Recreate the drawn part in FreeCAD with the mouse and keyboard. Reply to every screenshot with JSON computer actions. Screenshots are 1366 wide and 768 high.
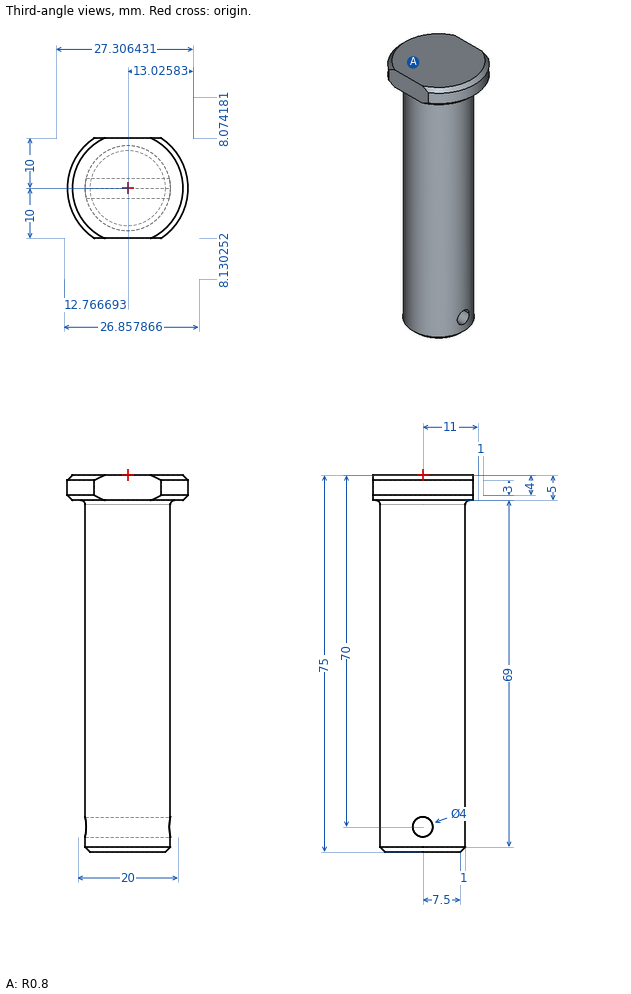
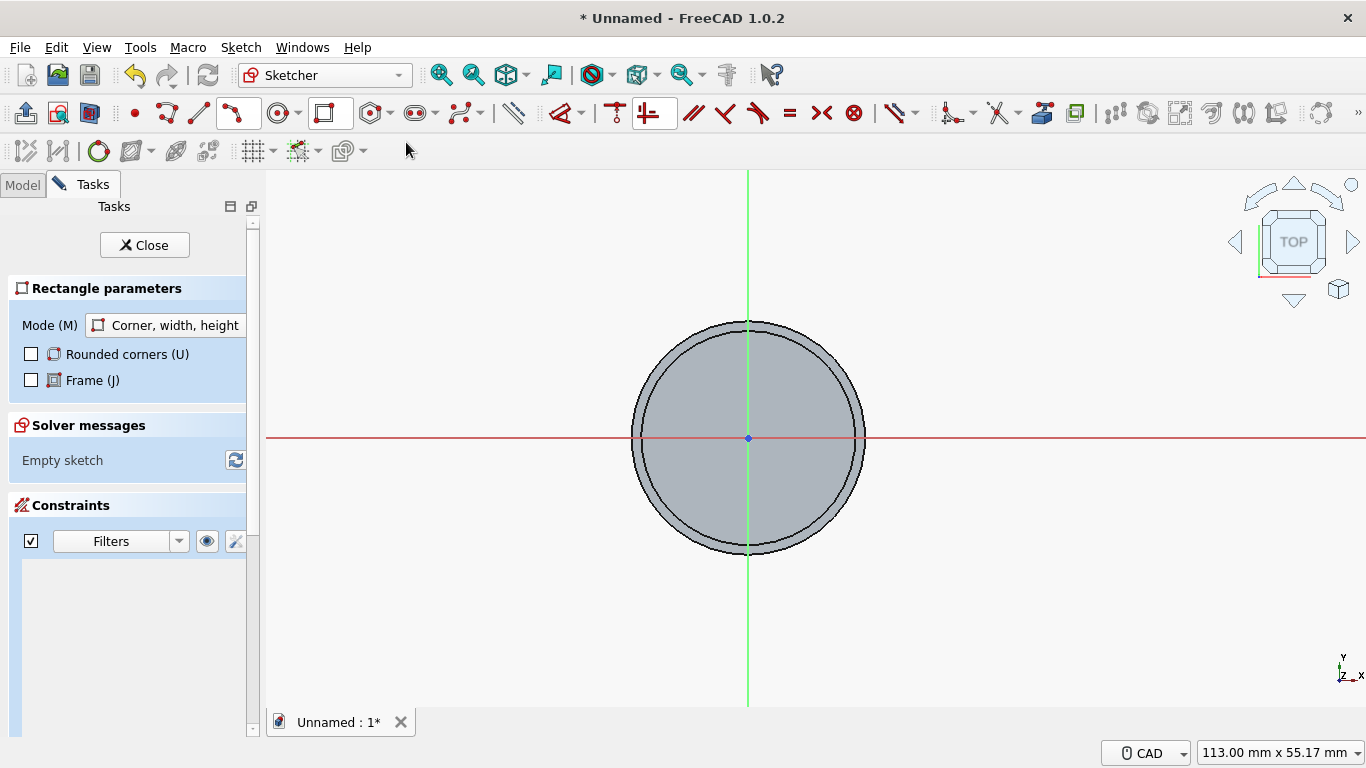
{"action": "left_click", "coordinate": [609, 262]}
{"action": "mouse_move", "coordinate": [875, 341]}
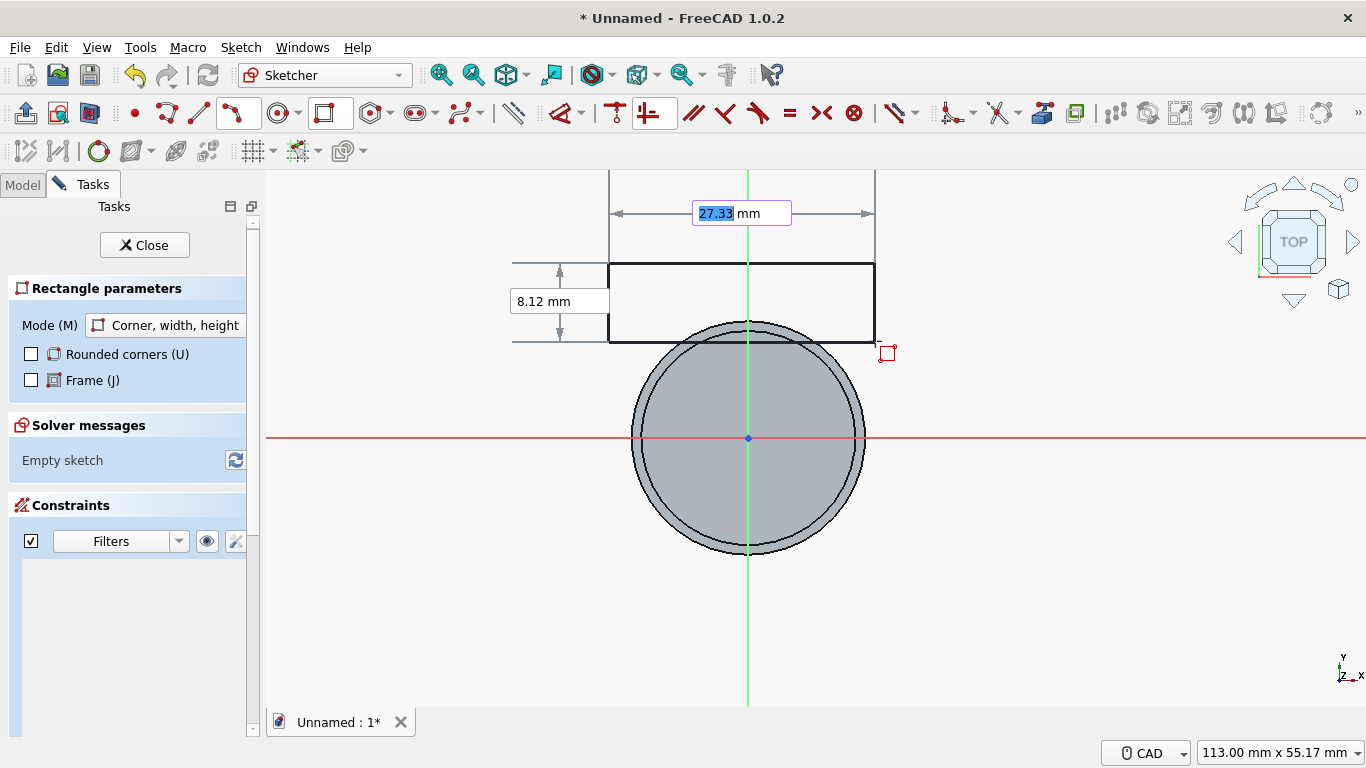
{"action": "type", "text": "27.306431"}
{"action": "key", "text": "Tab"}
{"action": "type", "text": "8.074181"}
{"action": "key", "text": "Return"}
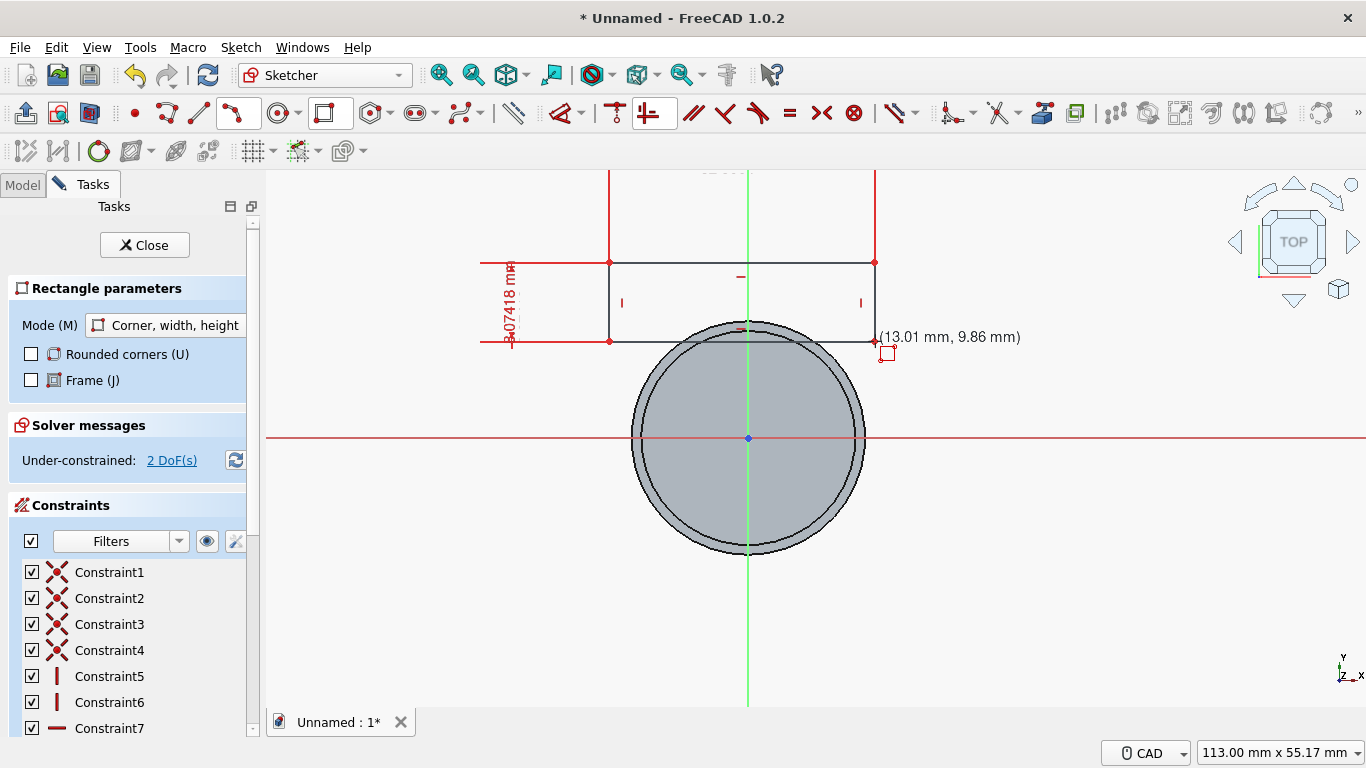
{"action": "left_click", "coordinate": [624, 535]}
{"action": "mouse_move", "coordinate": [885, 614]}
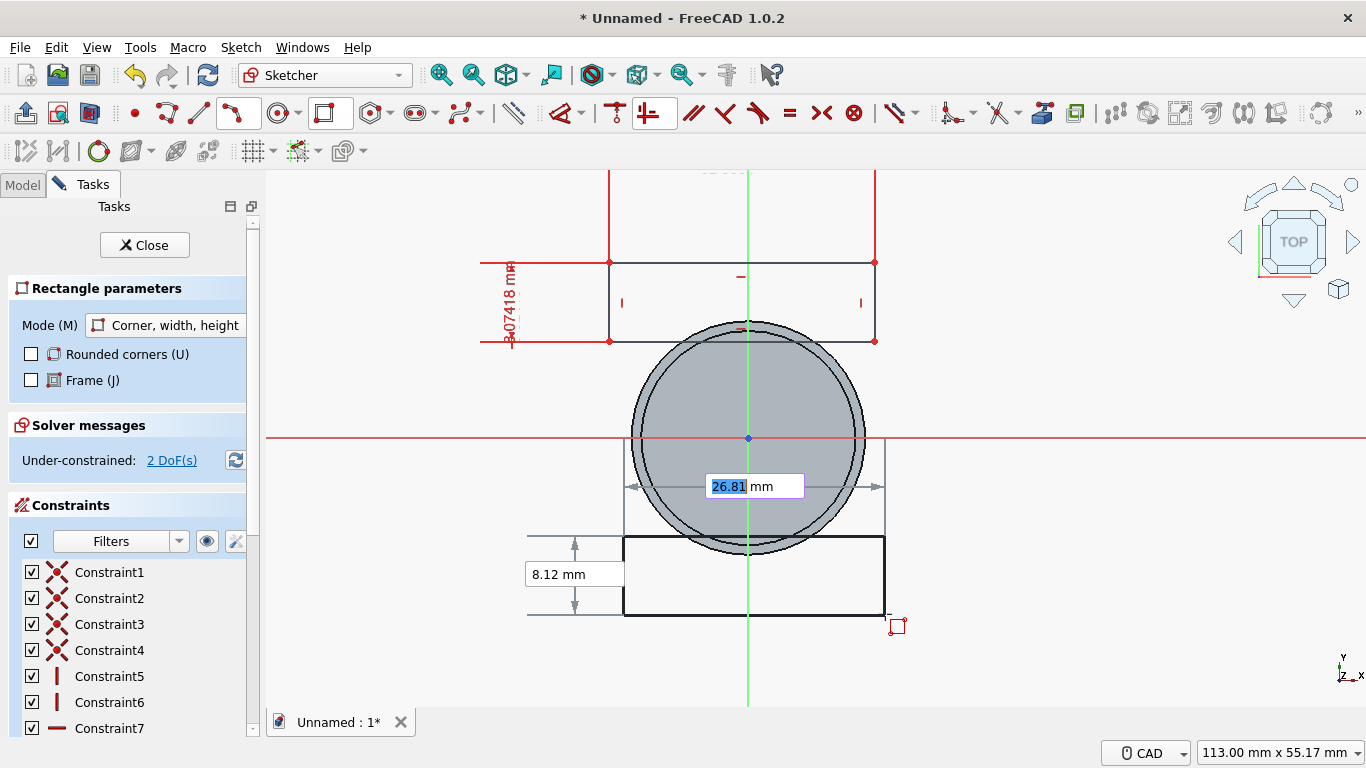
{"action": "type", "text": "26.857866"}
{"action": "key", "text": "Tab"}
{"action": "type", "text": "8.130252"}
{"action": "key", "text": "Return"}
{"action": "key", "text": "Escape"}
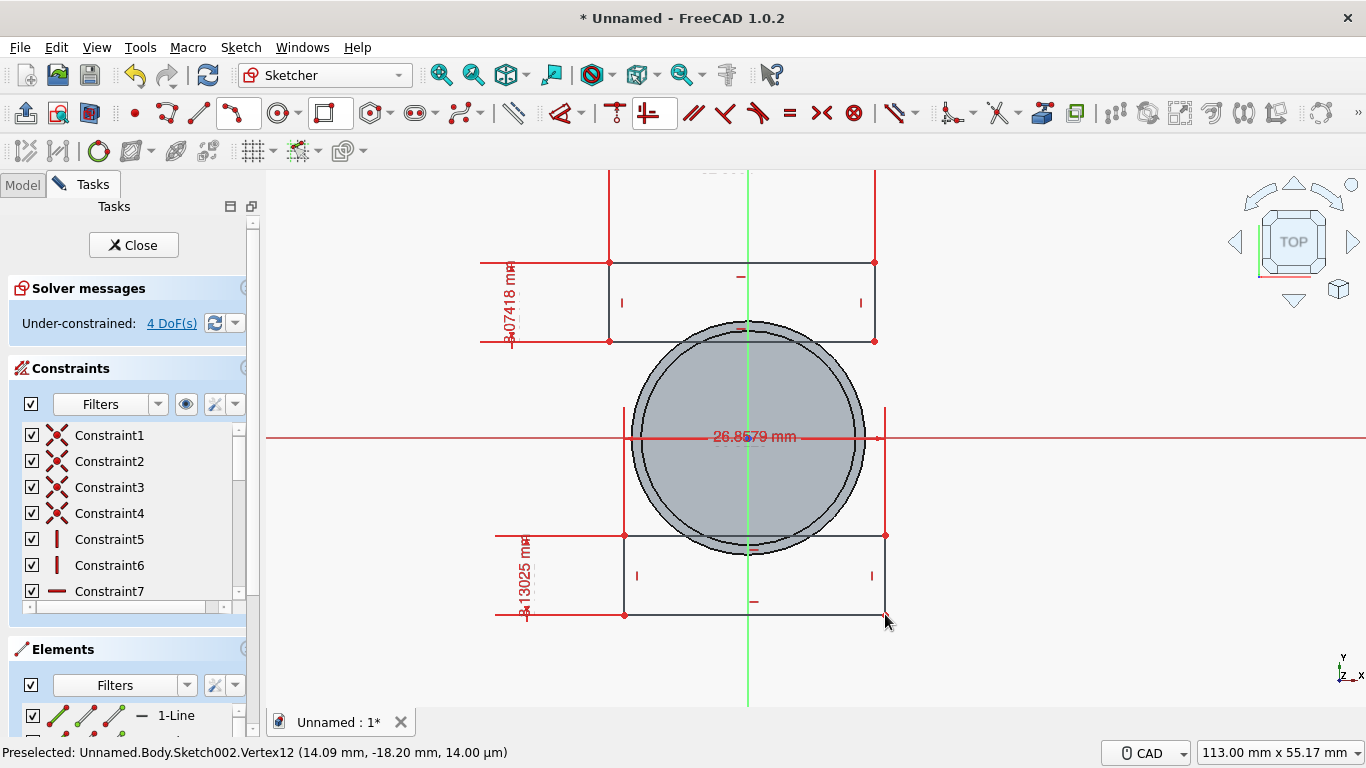
{"action": "left_click", "coordinate": [560, 114]}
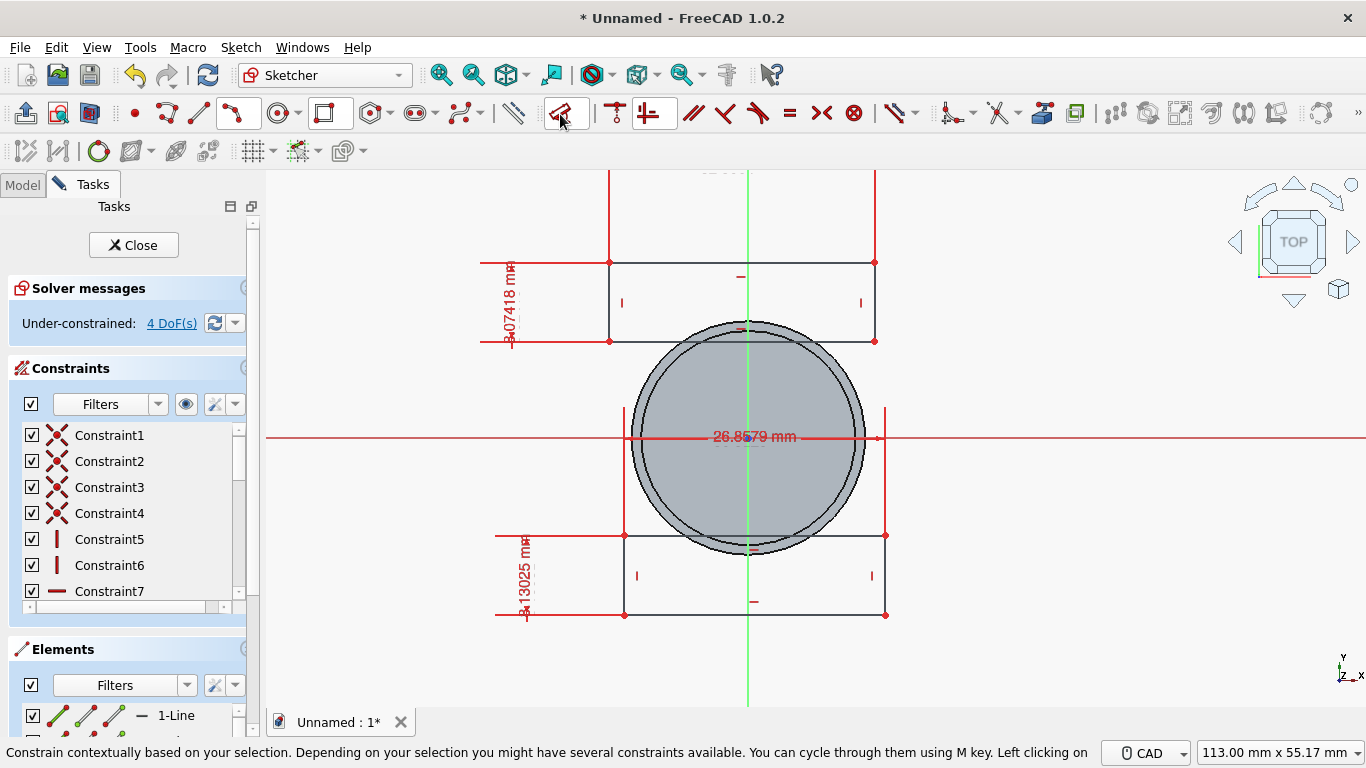
{"action": "left_click", "coordinate": [609, 342]}
{"action": "left_click", "coordinate": [575, 390]}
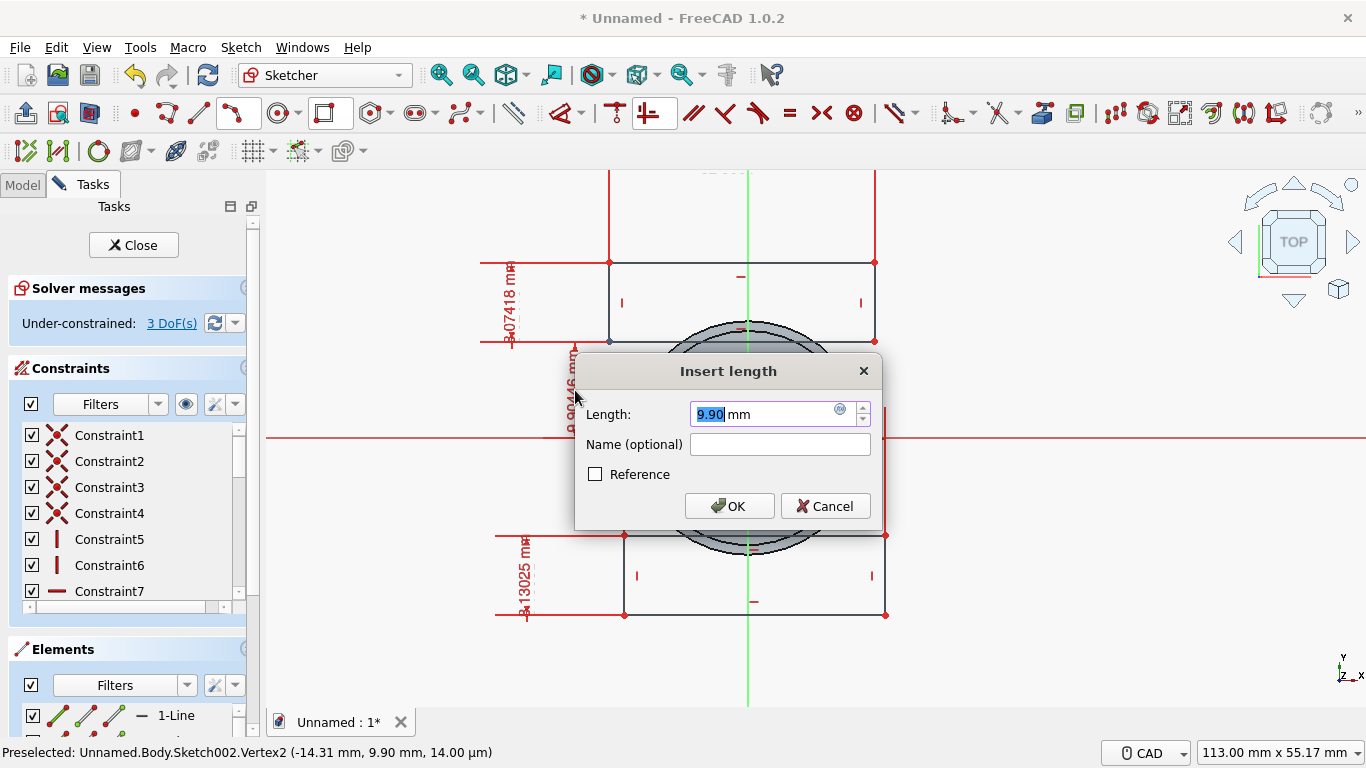
{"action": "type", "text": "10"}
{"action": "key", "text": "Return"}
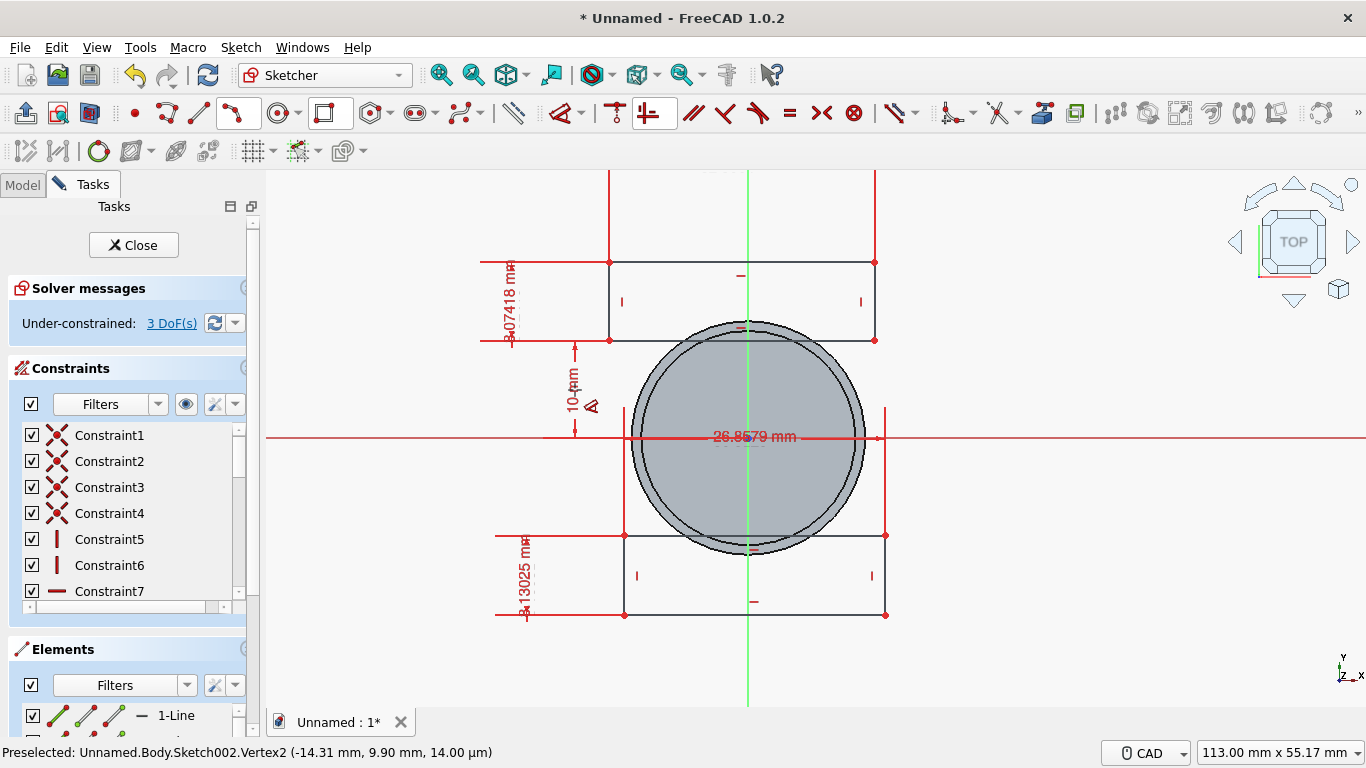
{"action": "left_click", "coordinate": [624, 536]}
{"action": "left_click", "coordinate": [590, 487]}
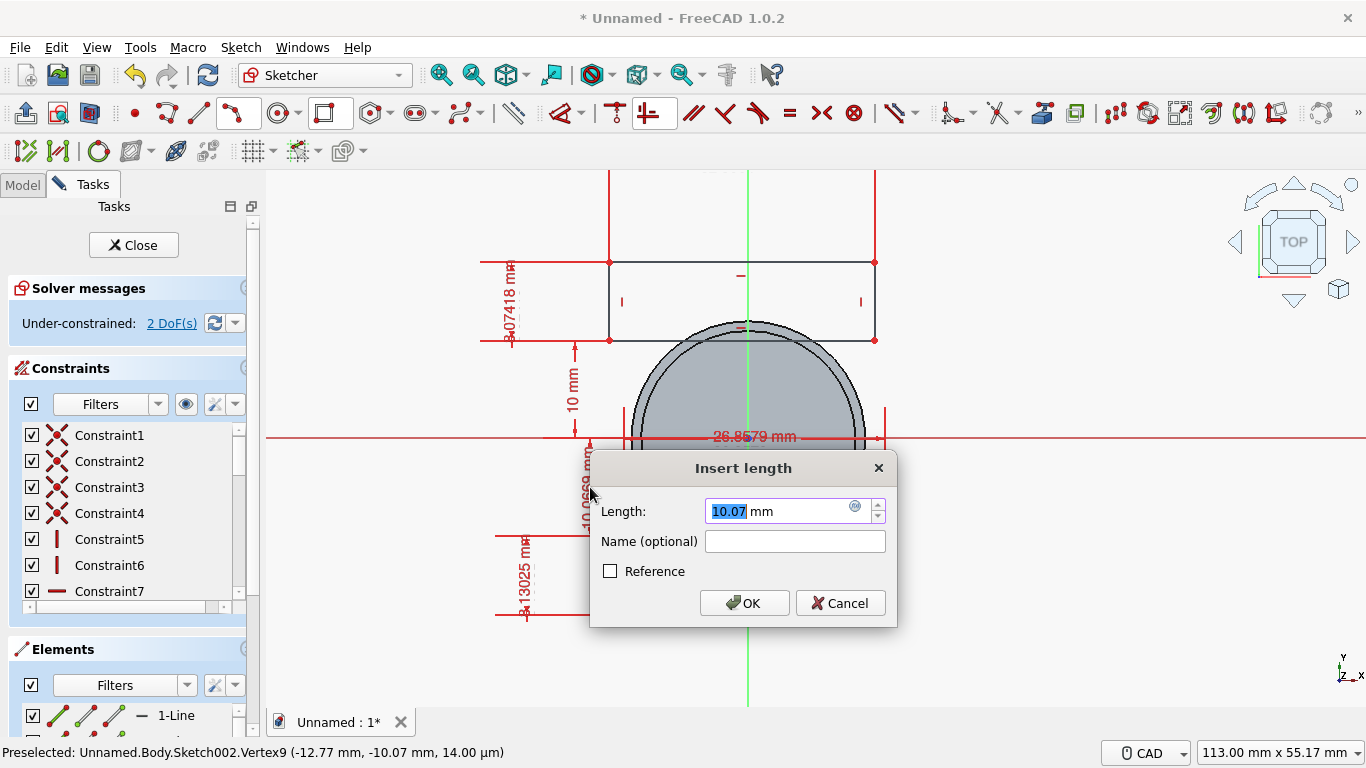
{"action": "type", "text": "10"}
{"action": "key", "text": "Return"}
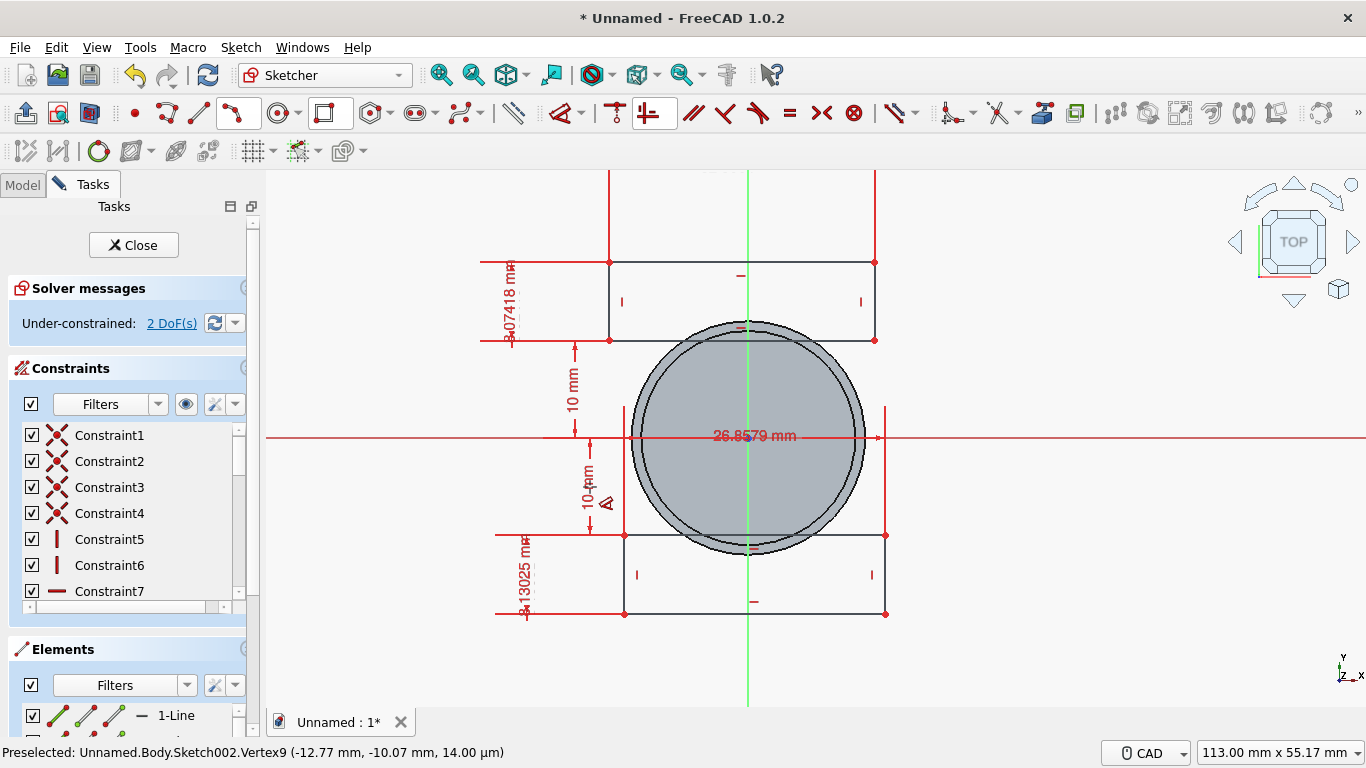
{"action": "left_click", "coordinate": [875, 341]}
{"action": "left_click", "coordinate": [812, 307]}